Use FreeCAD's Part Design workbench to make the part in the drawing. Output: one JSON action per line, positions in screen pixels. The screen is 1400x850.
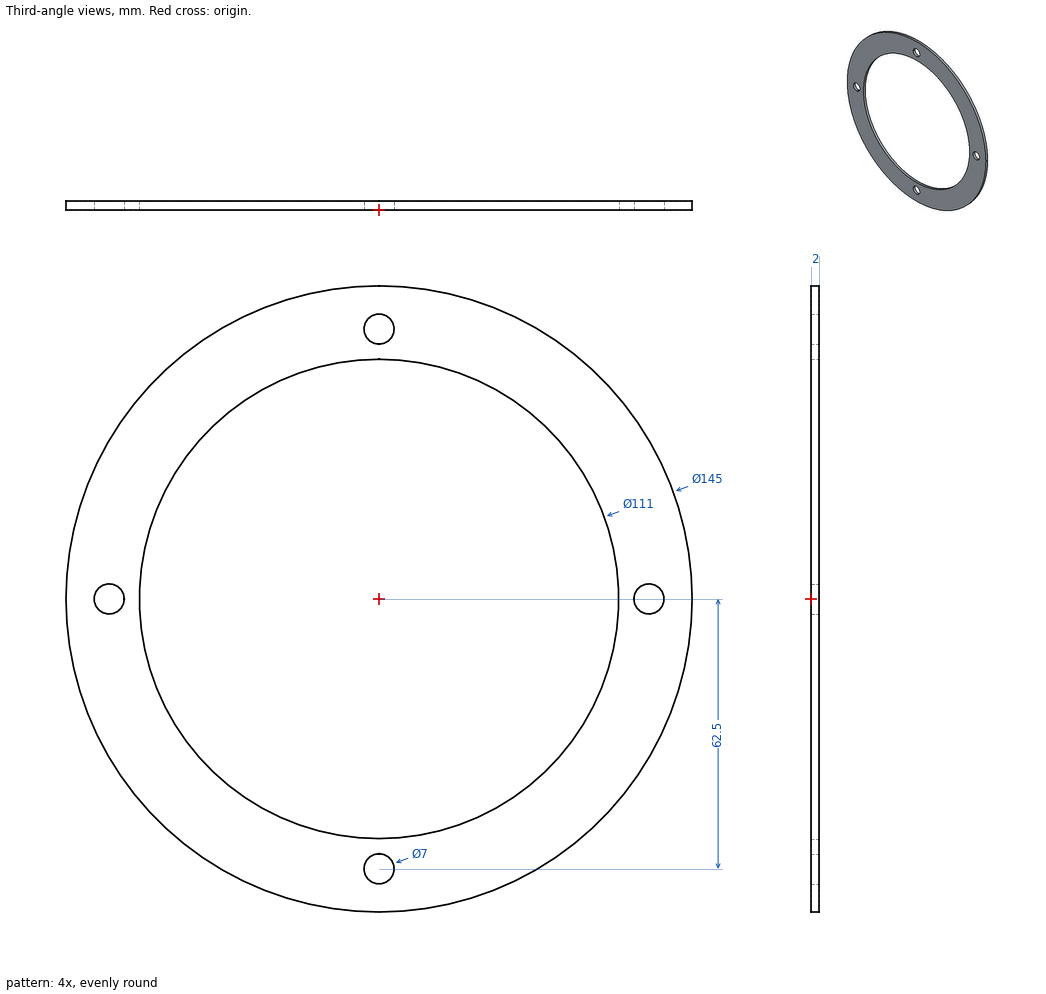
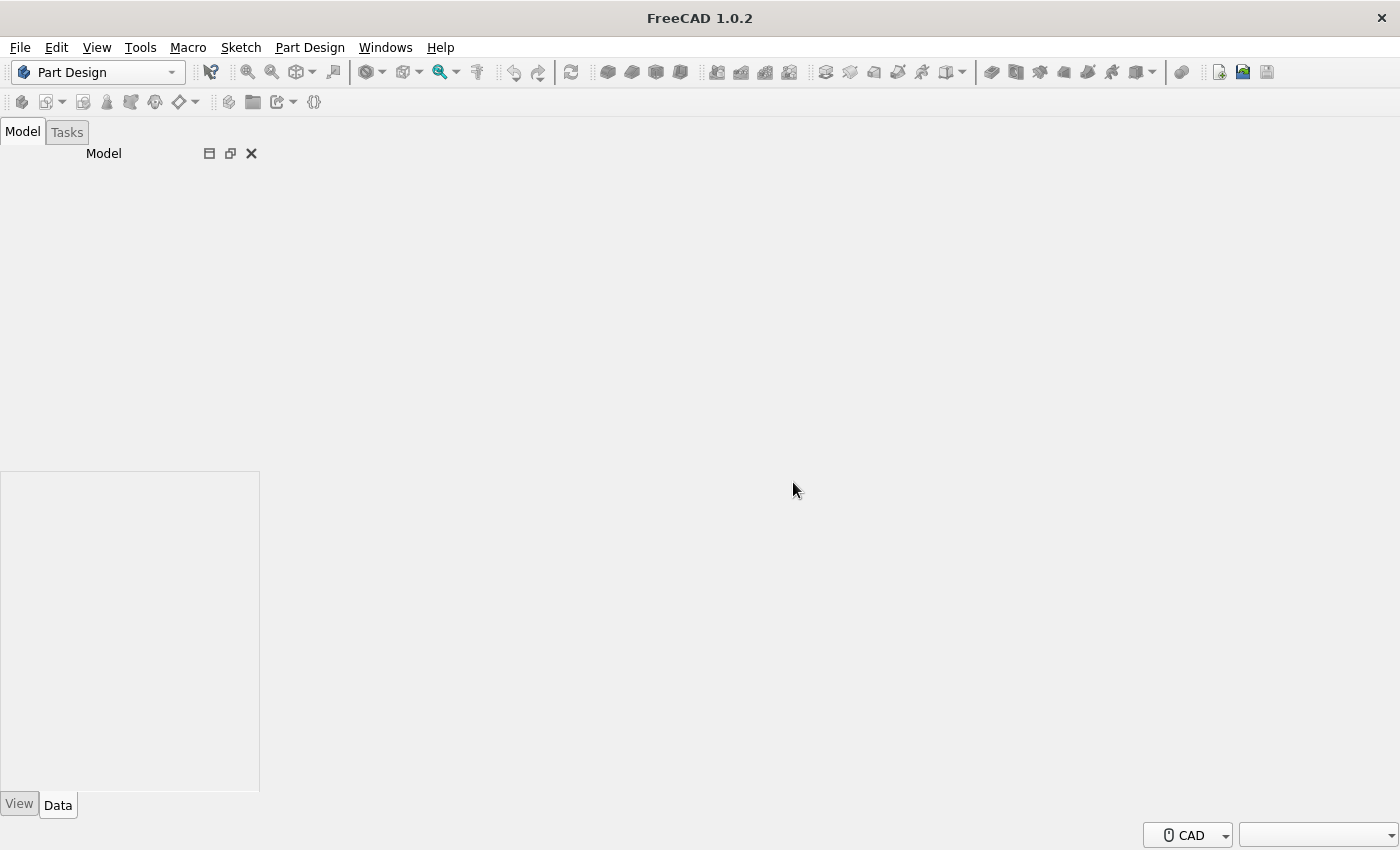
{"action": "left_click", "coordinate": [1220, 72]}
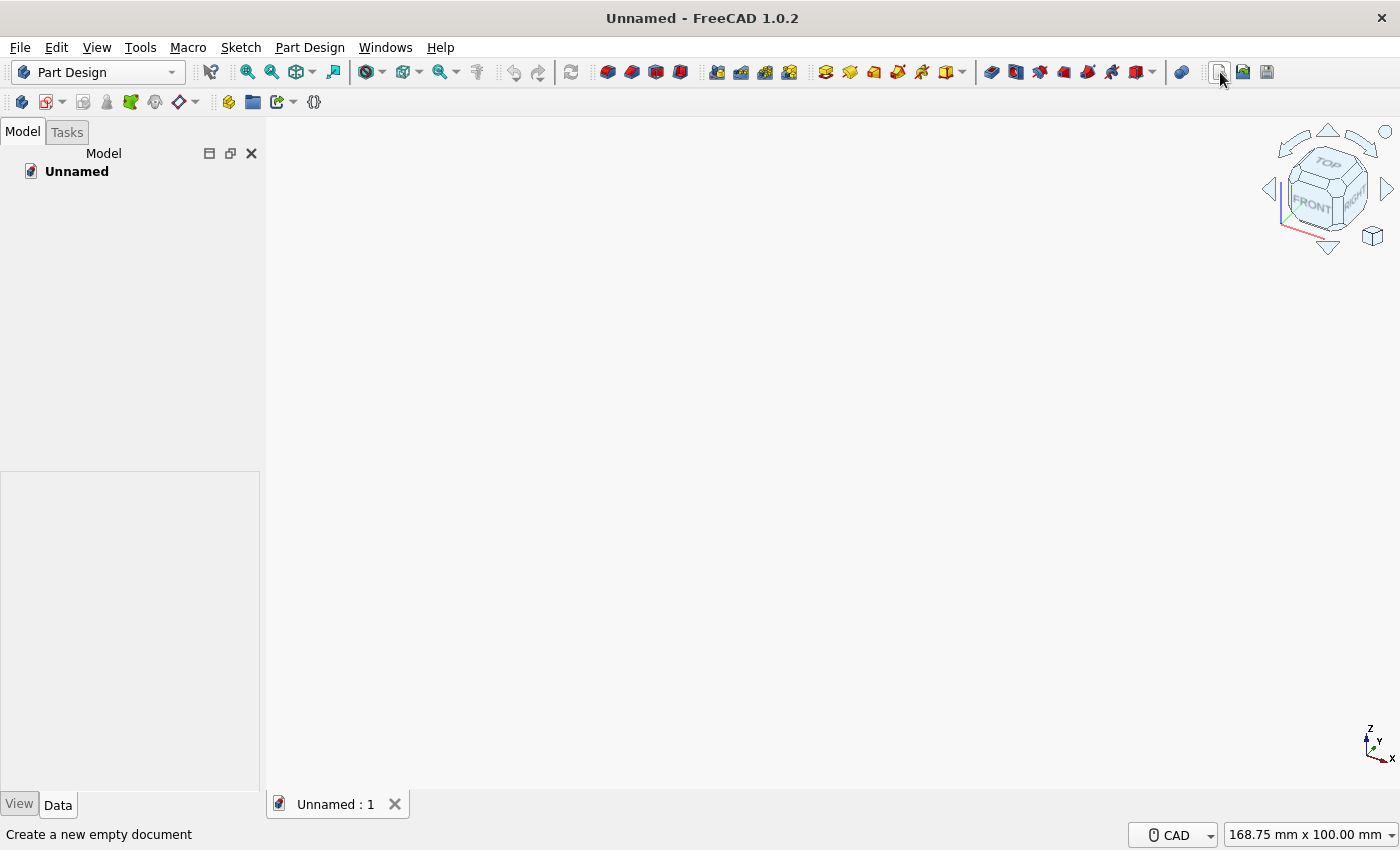
{"action": "left_click", "coordinate": [46, 102]}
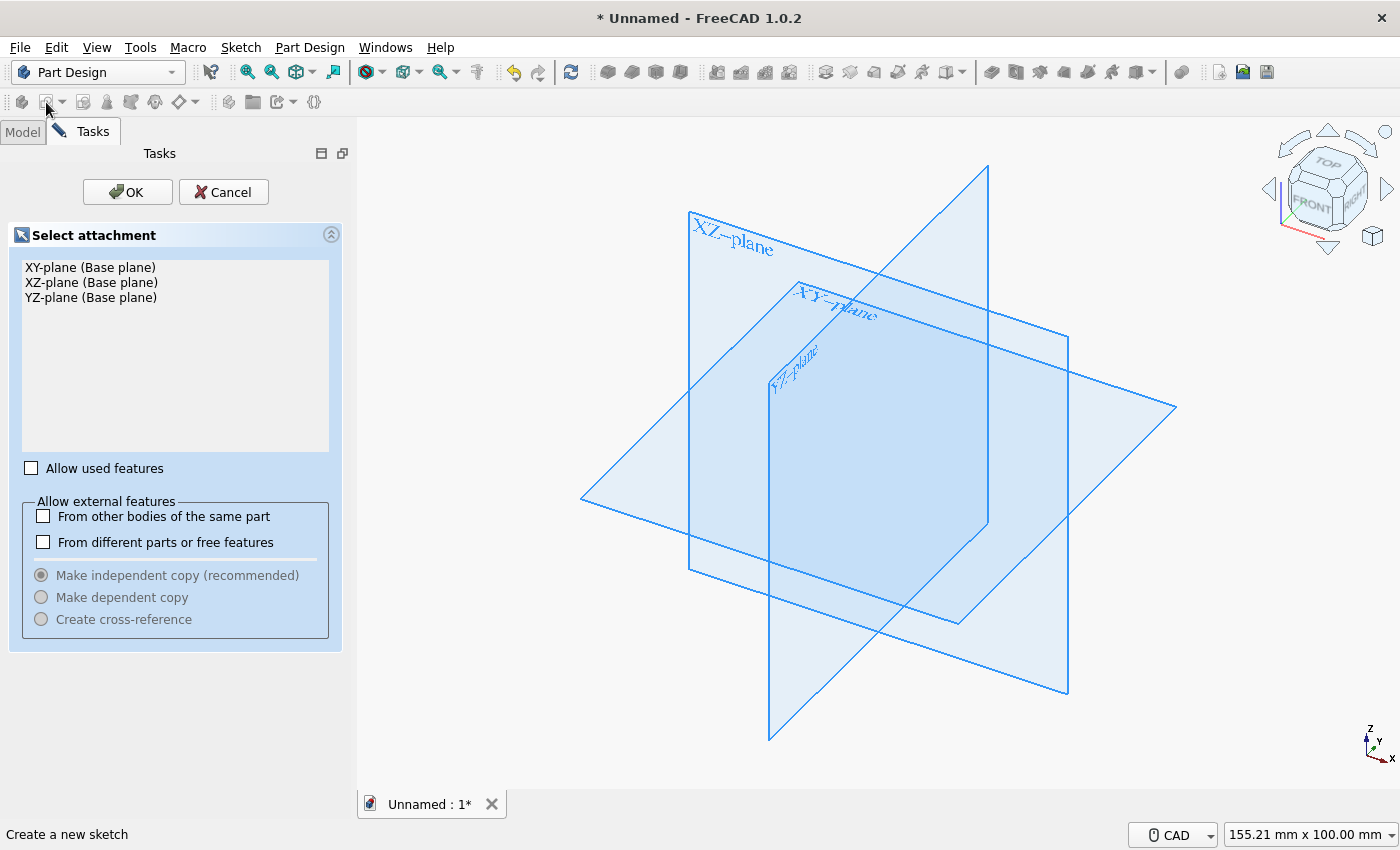
{"action": "left_click", "coordinate": [82, 282]}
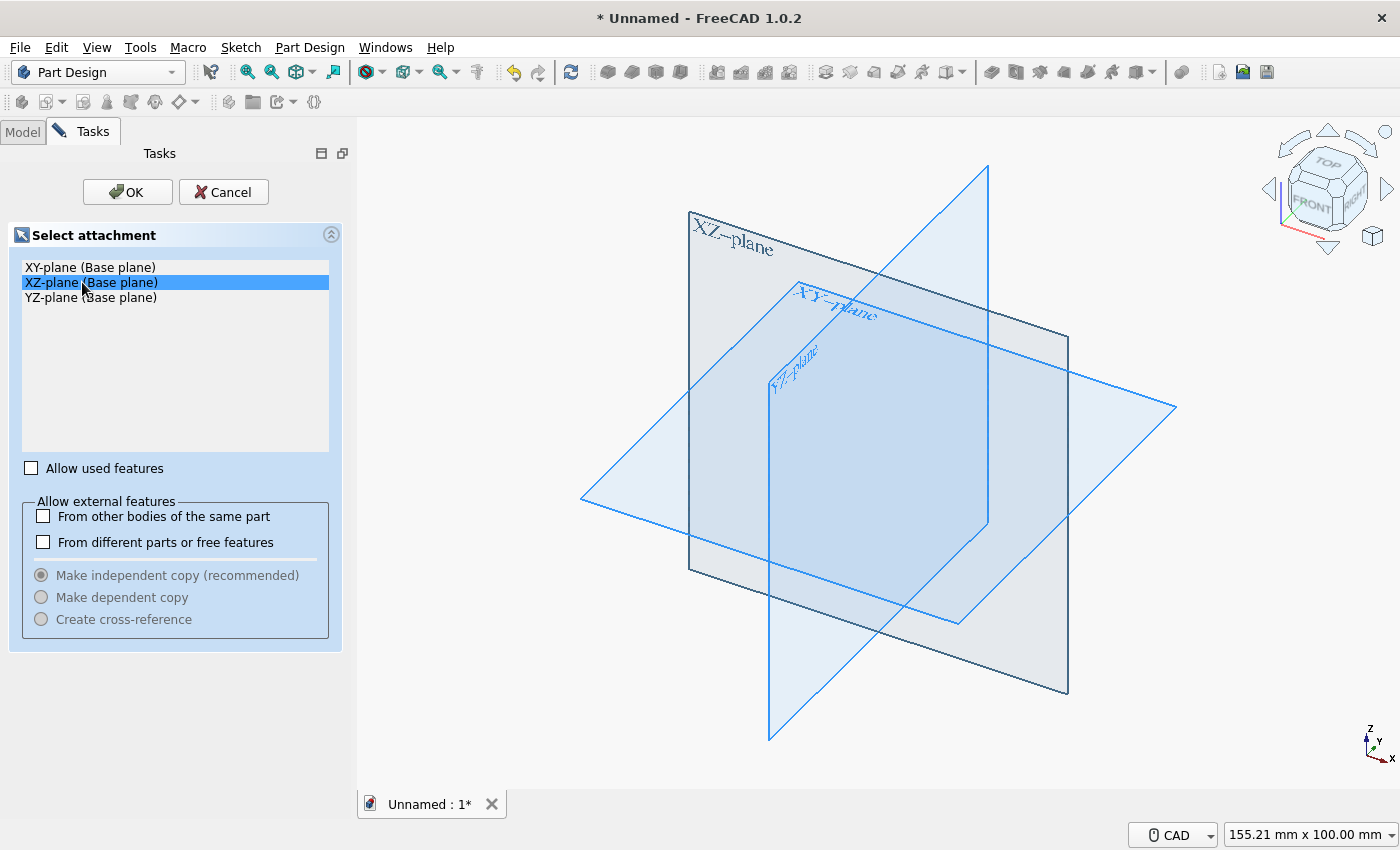
{"action": "left_click", "coordinate": [128, 192]}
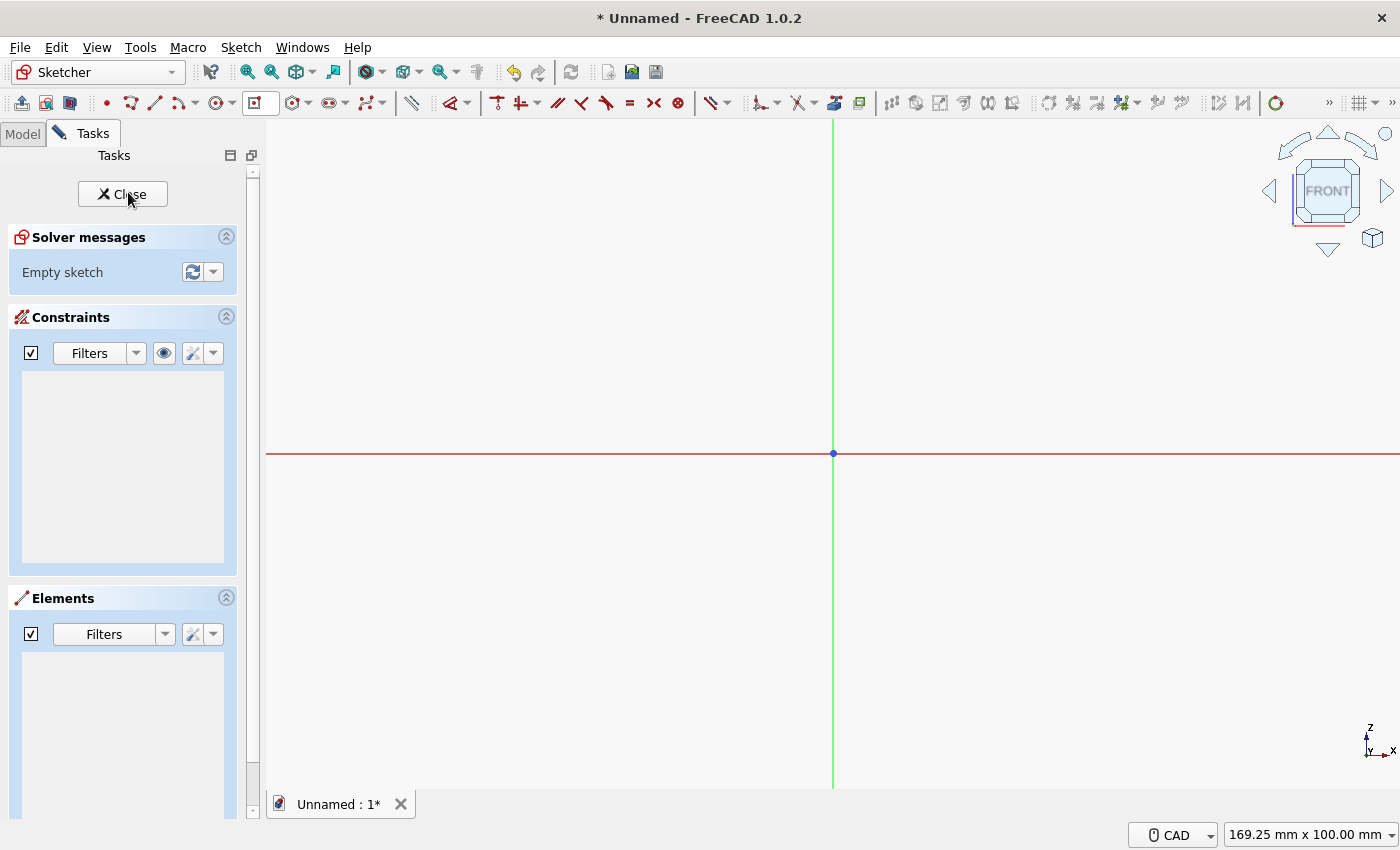
{"action": "scroll", "coordinate": [709, 454], "scroll_direction": "down", "scroll_amount": 4}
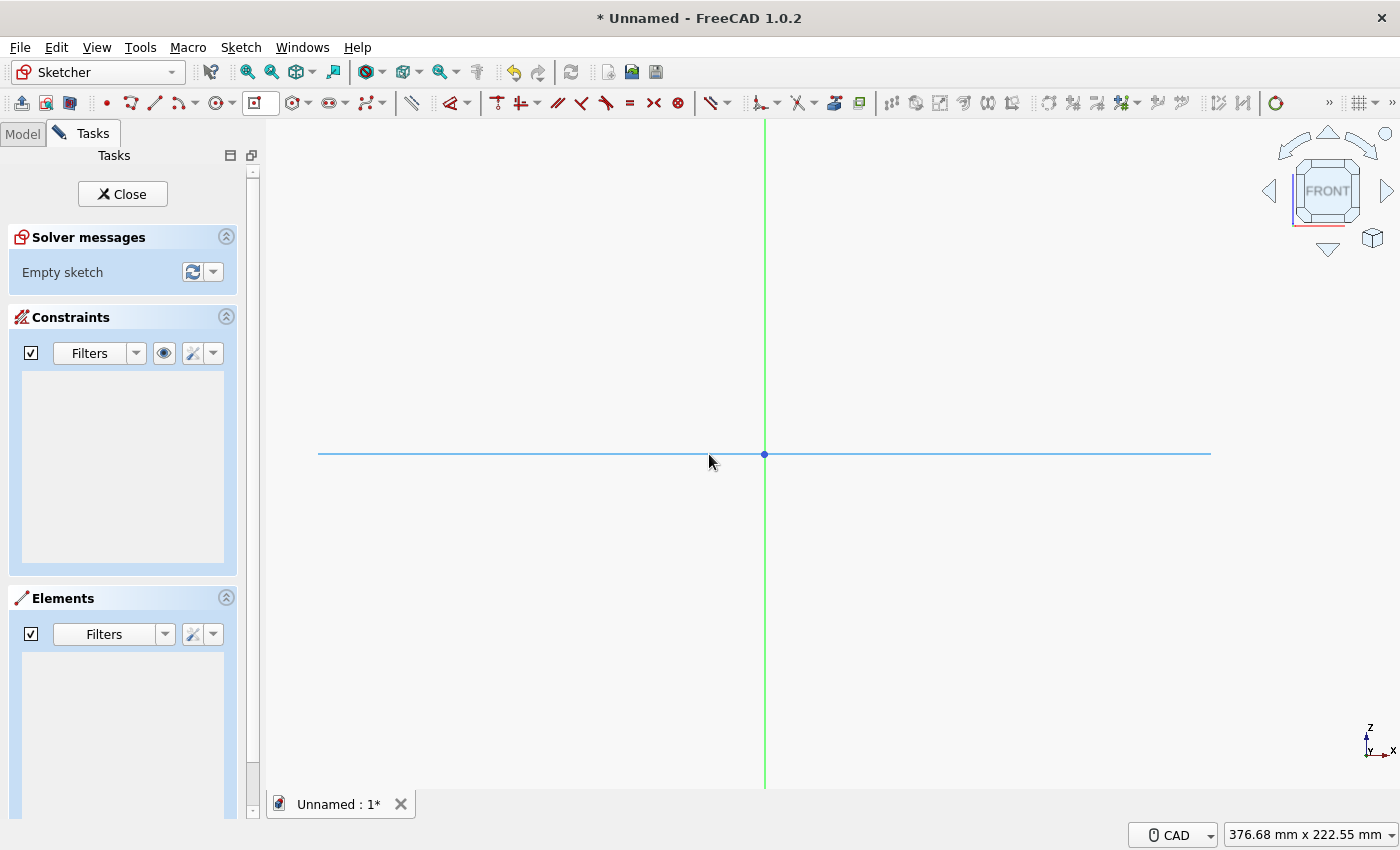
{"action": "left_click", "coordinate": [216, 104]}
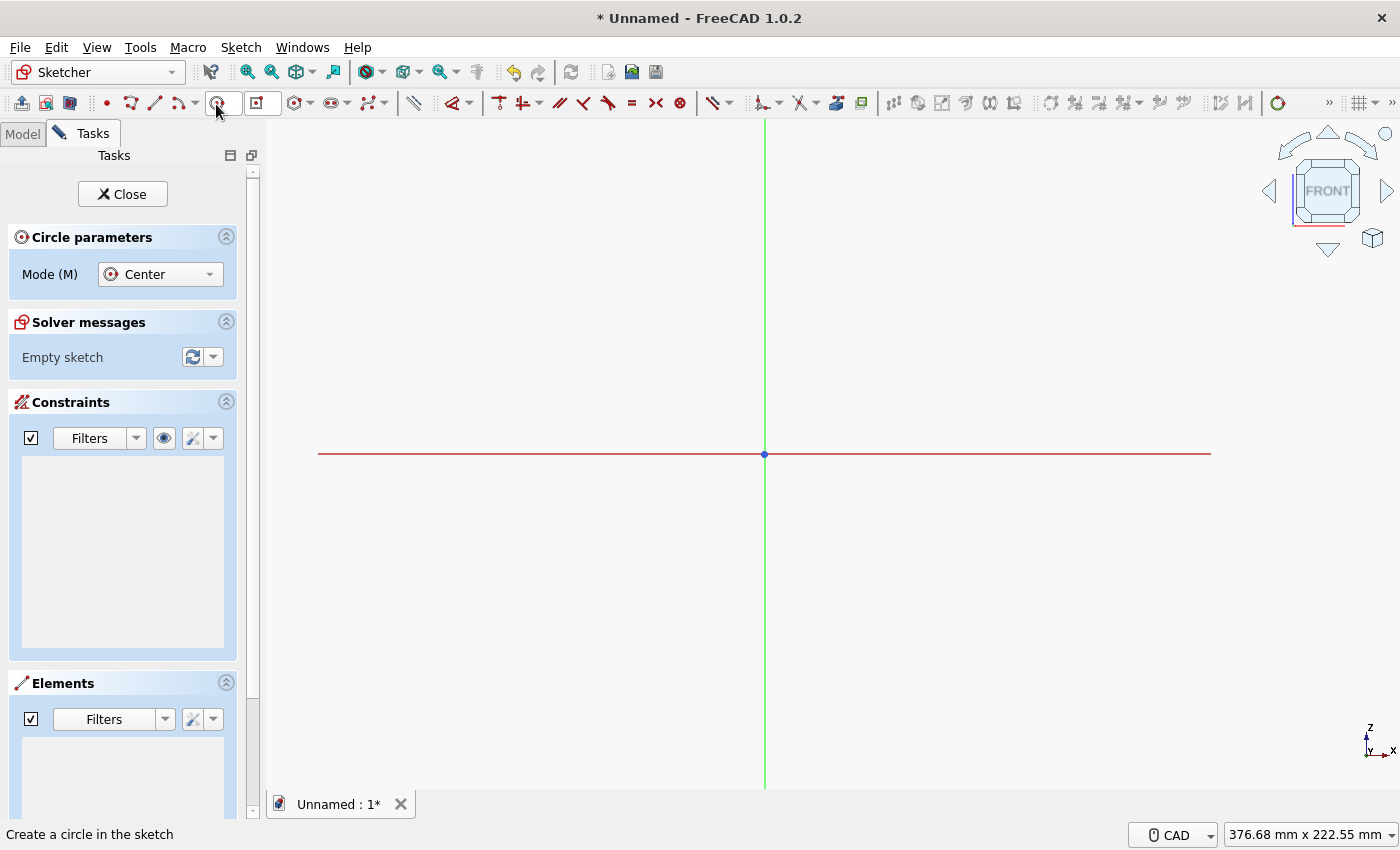
{"action": "left_click", "coordinate": [765, 454]}
{"action": "left_click", "coordinate": [919, 300]}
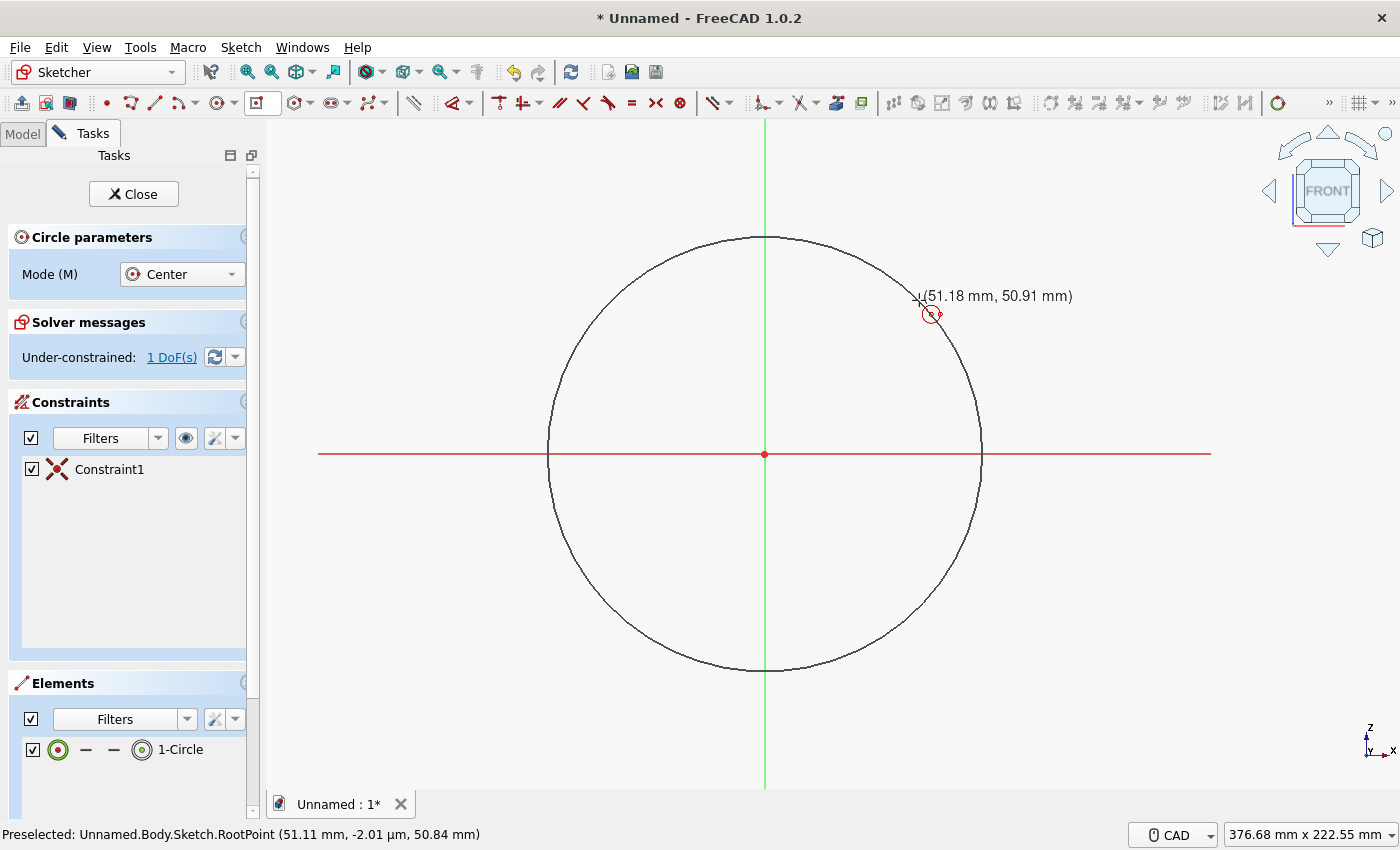
{"action": "left_click", "coordinate": [765, 454]}
{"action": "left_click", "coordinate": [883, 336]}
{"action": "key", "text": "Escape"}